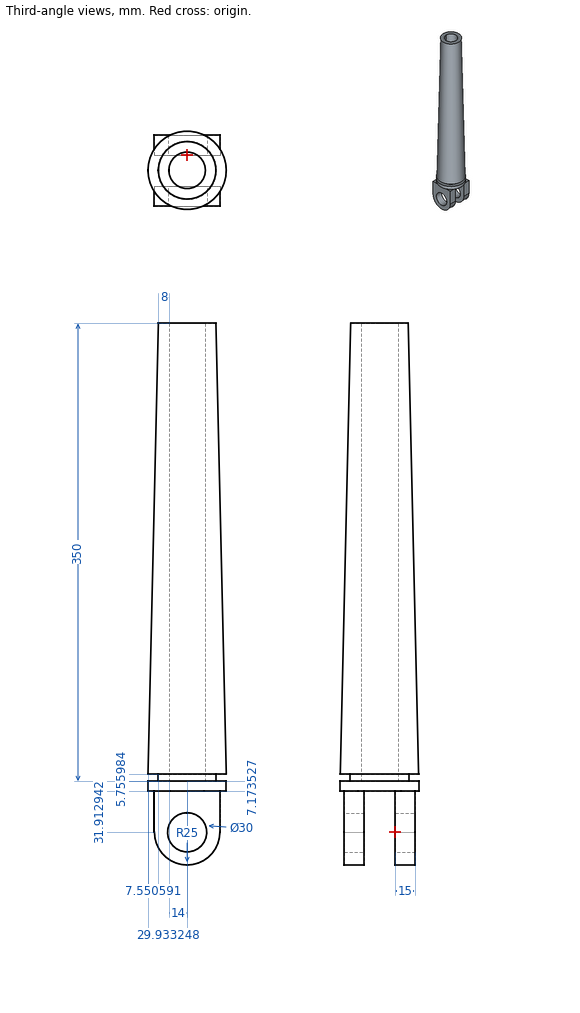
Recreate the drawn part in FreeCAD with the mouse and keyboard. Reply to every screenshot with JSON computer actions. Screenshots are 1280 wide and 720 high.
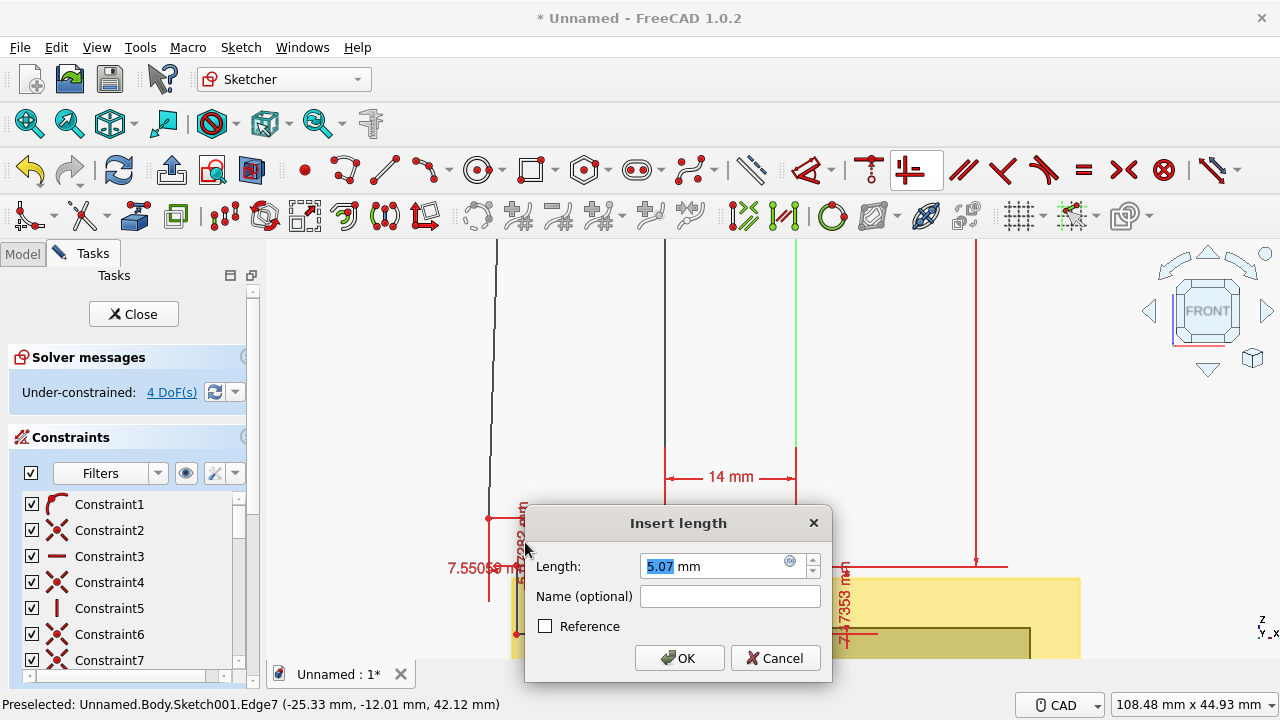
{"action": "type", "text": "5.755984"}
{"action": "key", "text": "Return"}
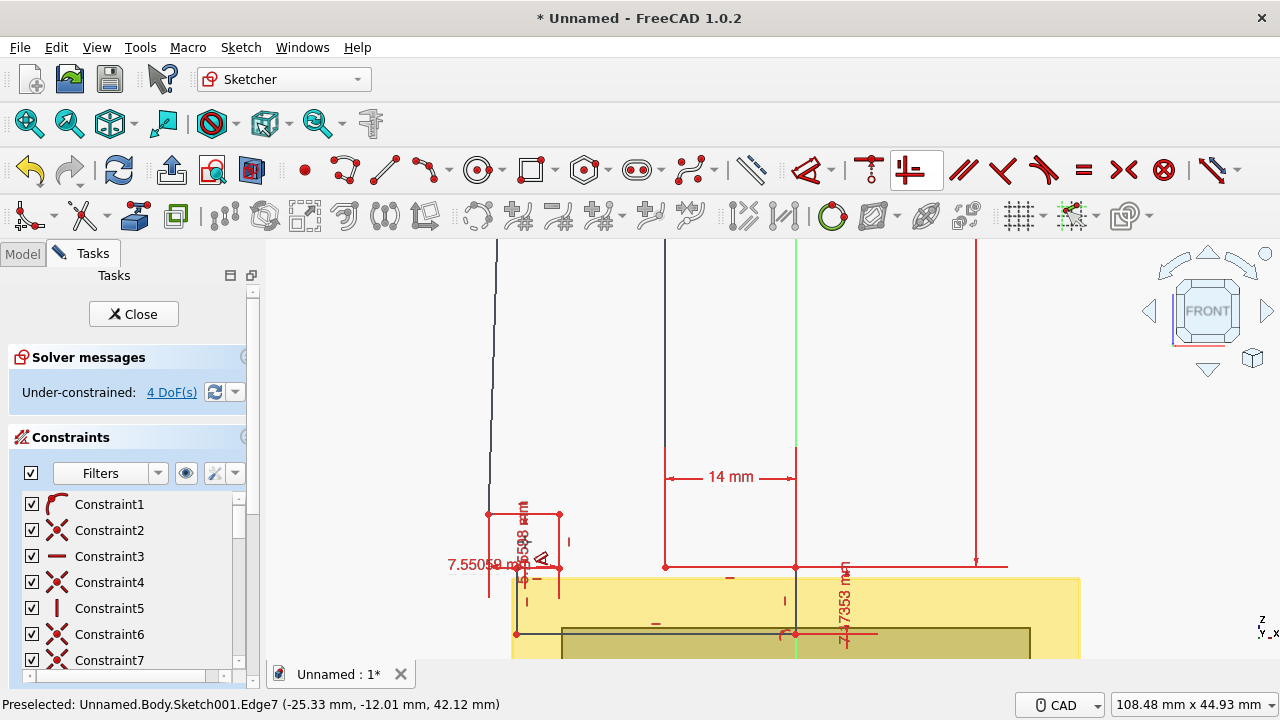
{"action": "left_click", "coordinate": [546, 568]}
{"action": "left_click", "coordinate": [538, 602]}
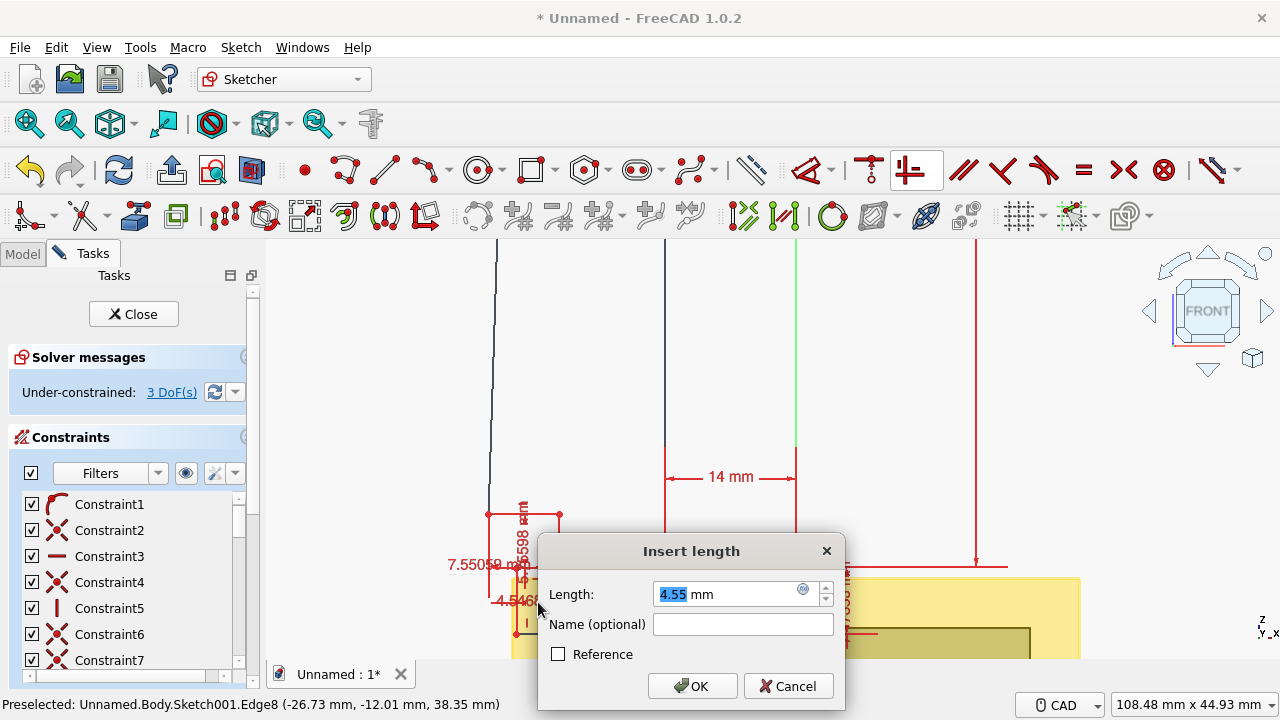
{"action": "type", "text": "7.550591"}
{"action": "key", "text": "Return"}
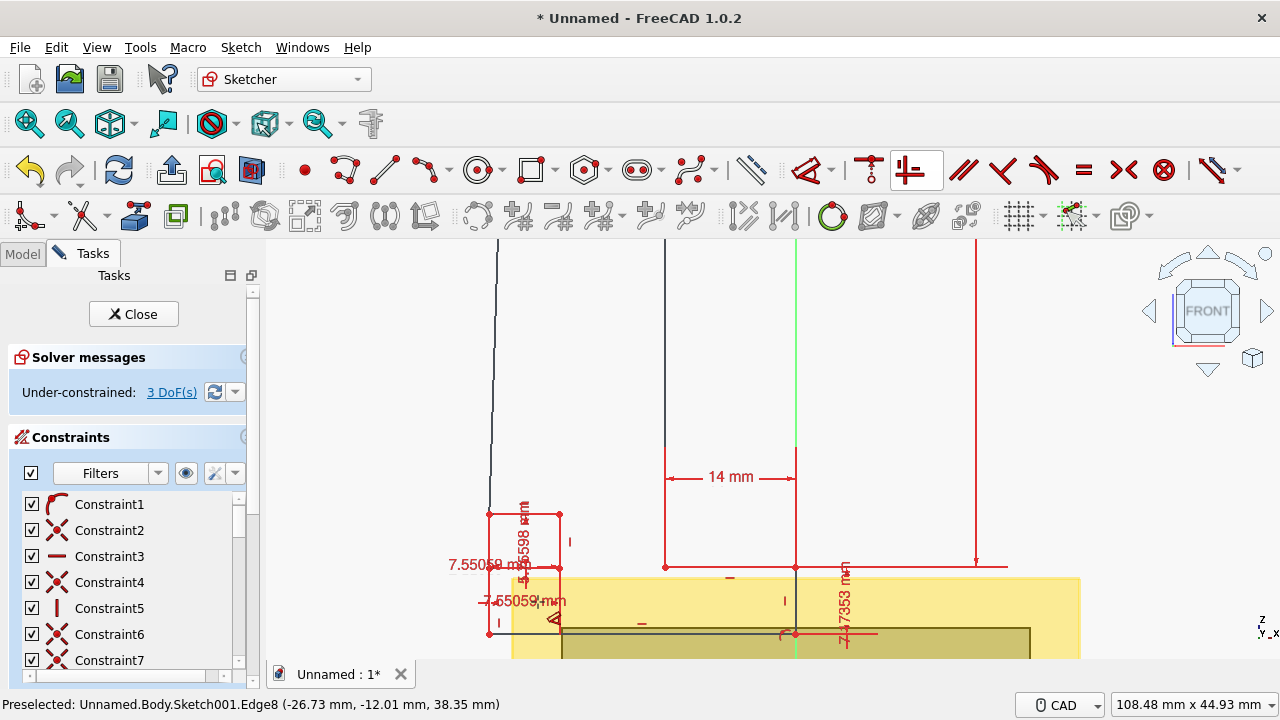
{"action": "left_click", "coordinate": [489, 588]}
{"action": "left_click", "coordinate": [455, 600]}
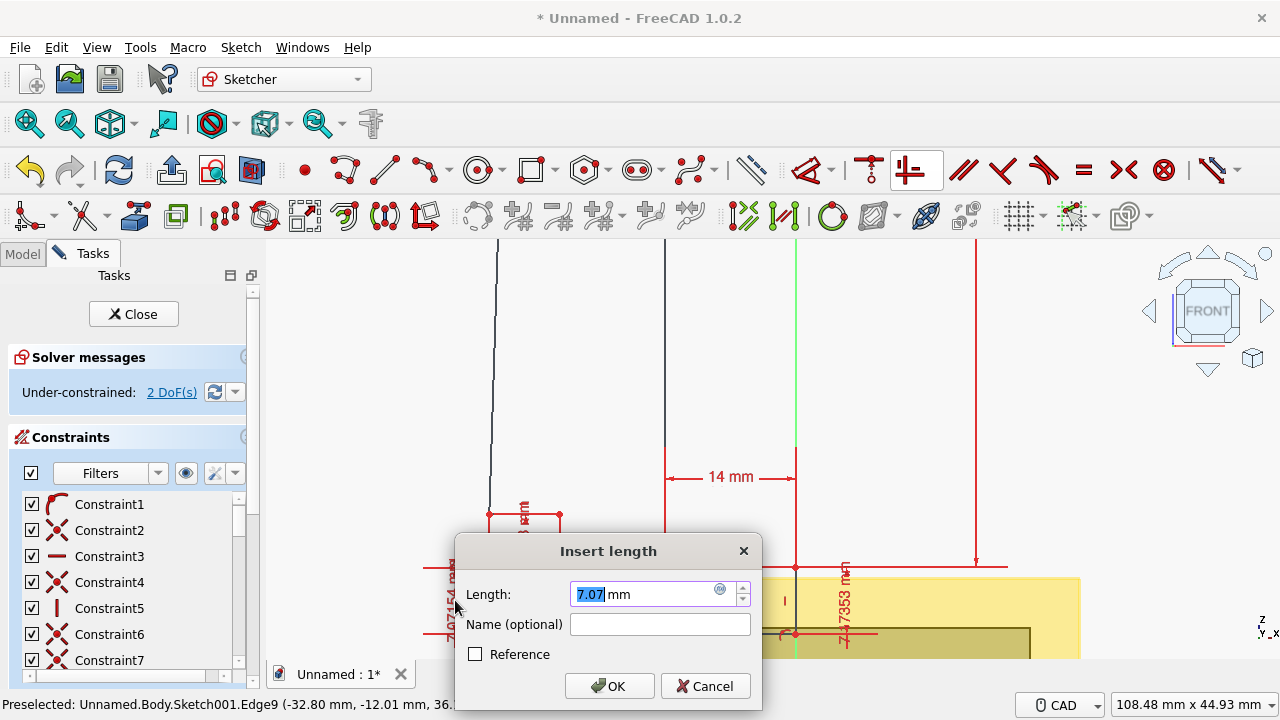
{"action": "type", "text": "7.173527"}
{"action": "key", "text": "Return"}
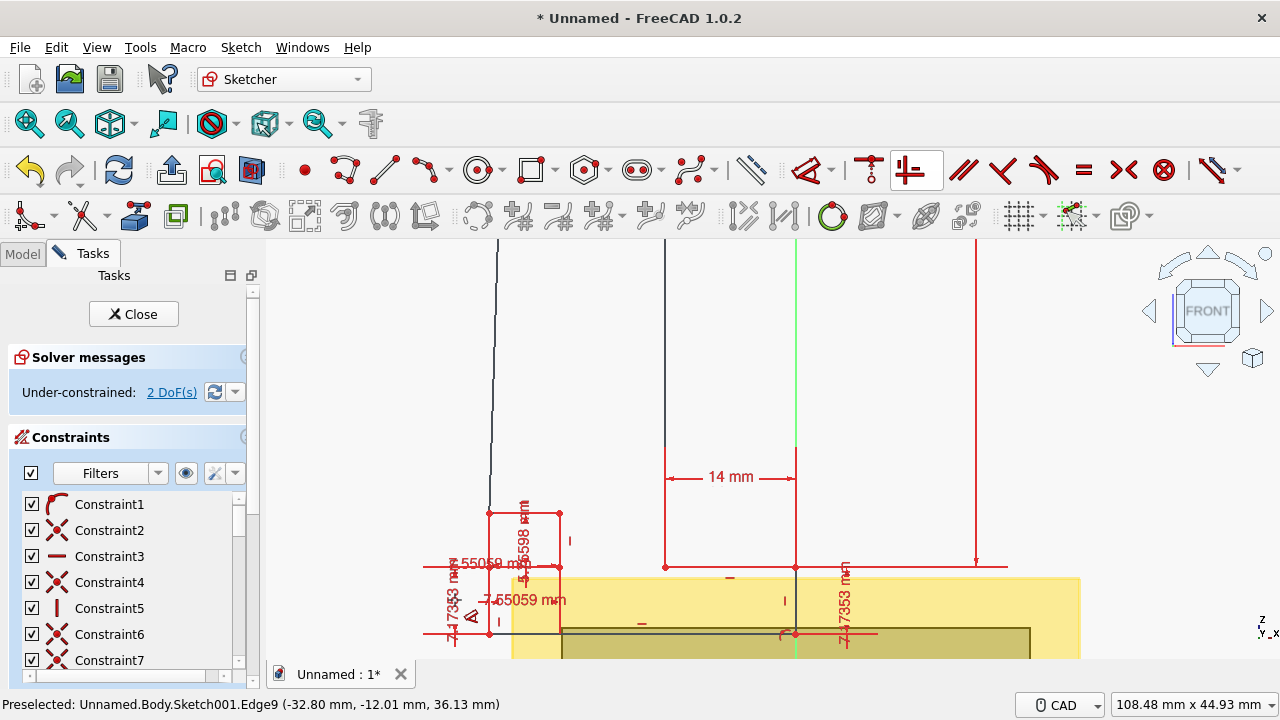
{"action": "scroll", "coordinate": [708, 557], "scroll_direction": "down", "scroll_amount": 13}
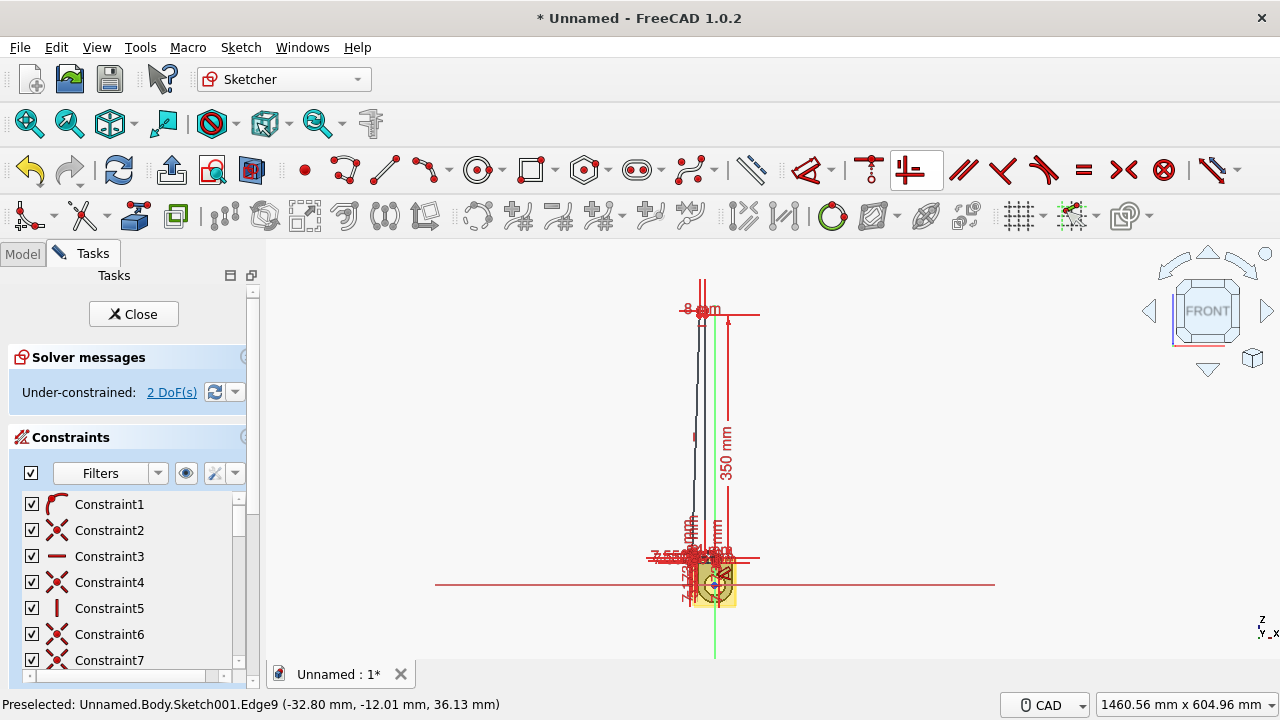
{"action": "scroll", "coordinate": [699, 563], "scroll_direction": "up", "scroll_amount": 5}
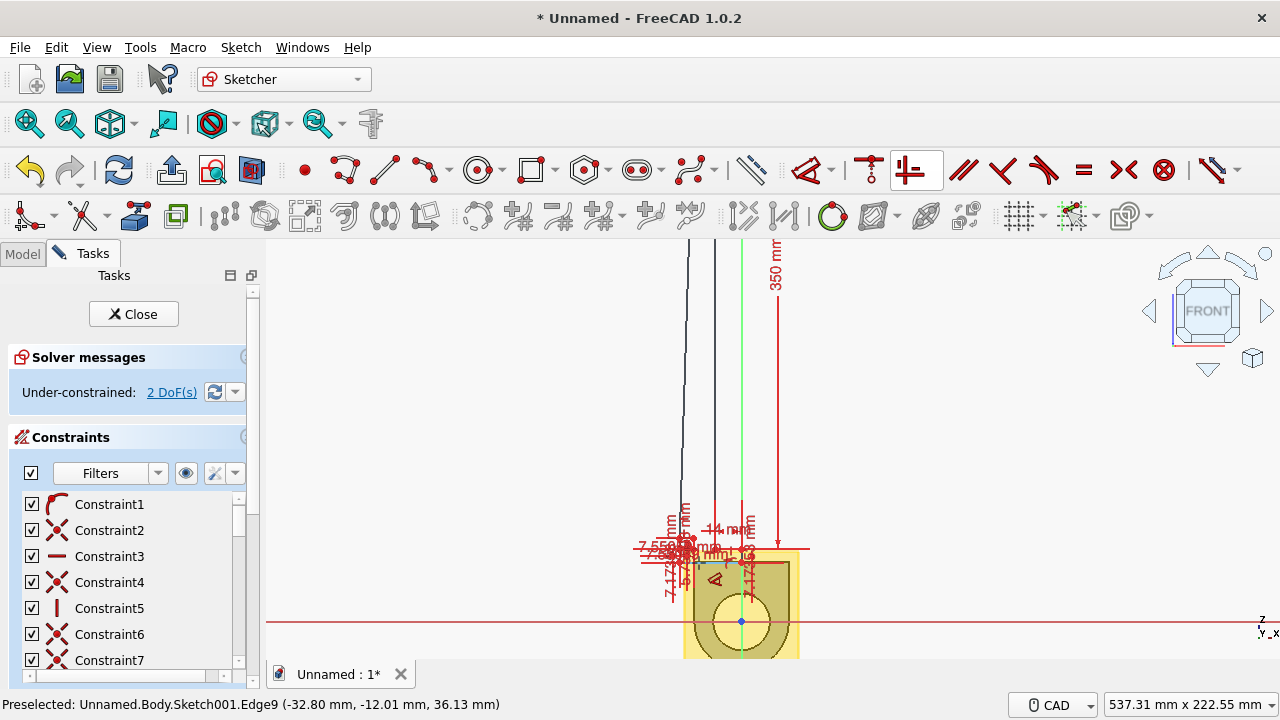
{"action": "left_click", "coordinate": [698, 563]}
{"action": "left_click", "coordinate": [711, 597]}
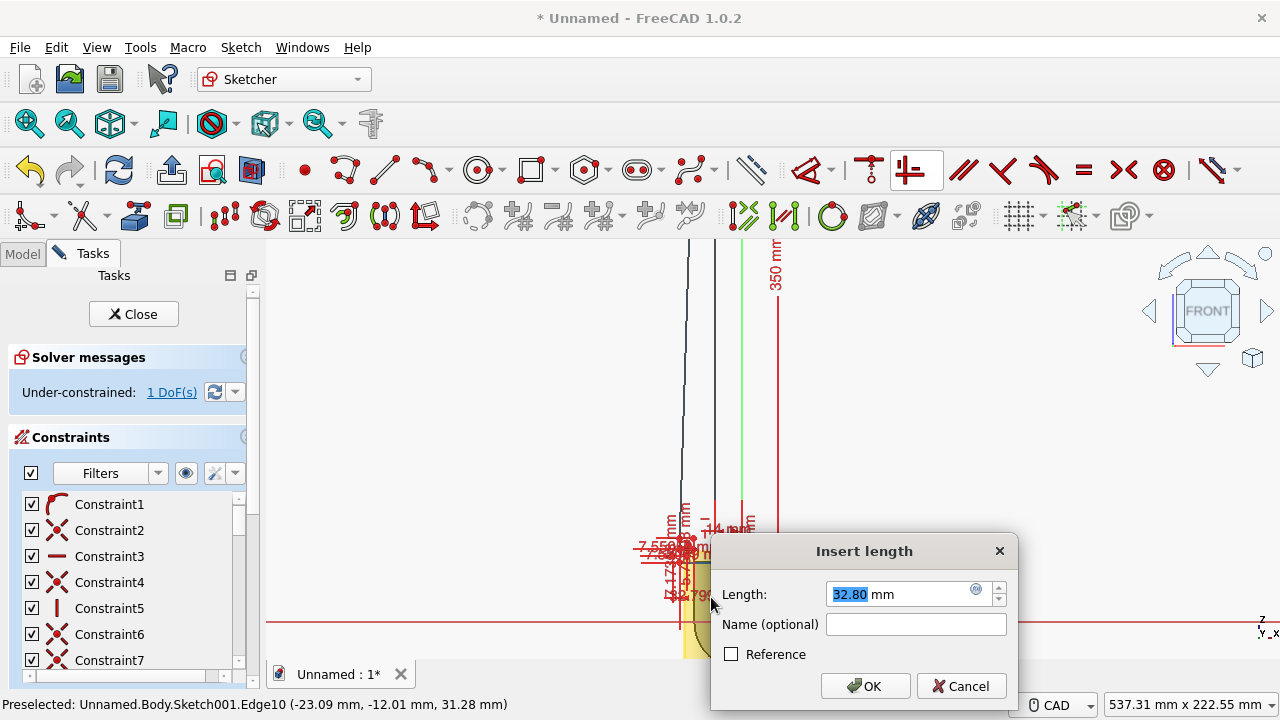
{"action": "type", "text": "29.933248"}
{"action": "key", "text": "Return"}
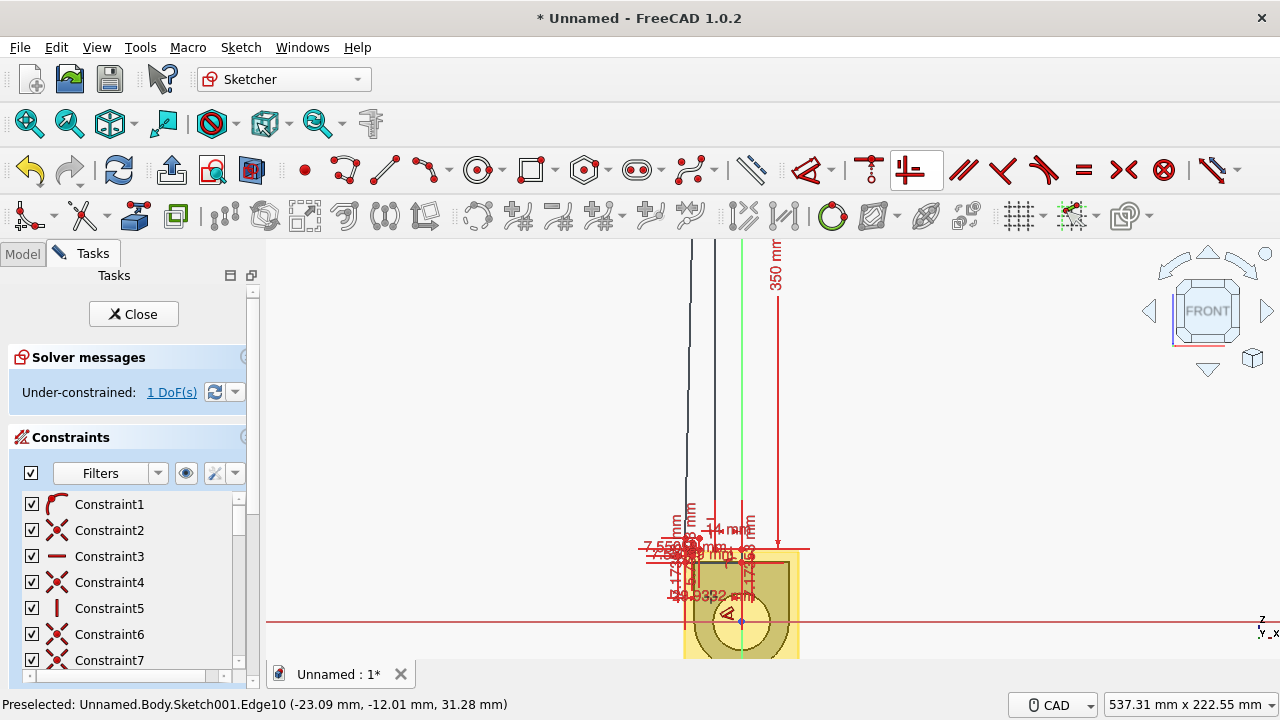
{"action": "left_click", "coordinate": [742, 563]}
{"action": "left_click", "coordinate": [800, 592]}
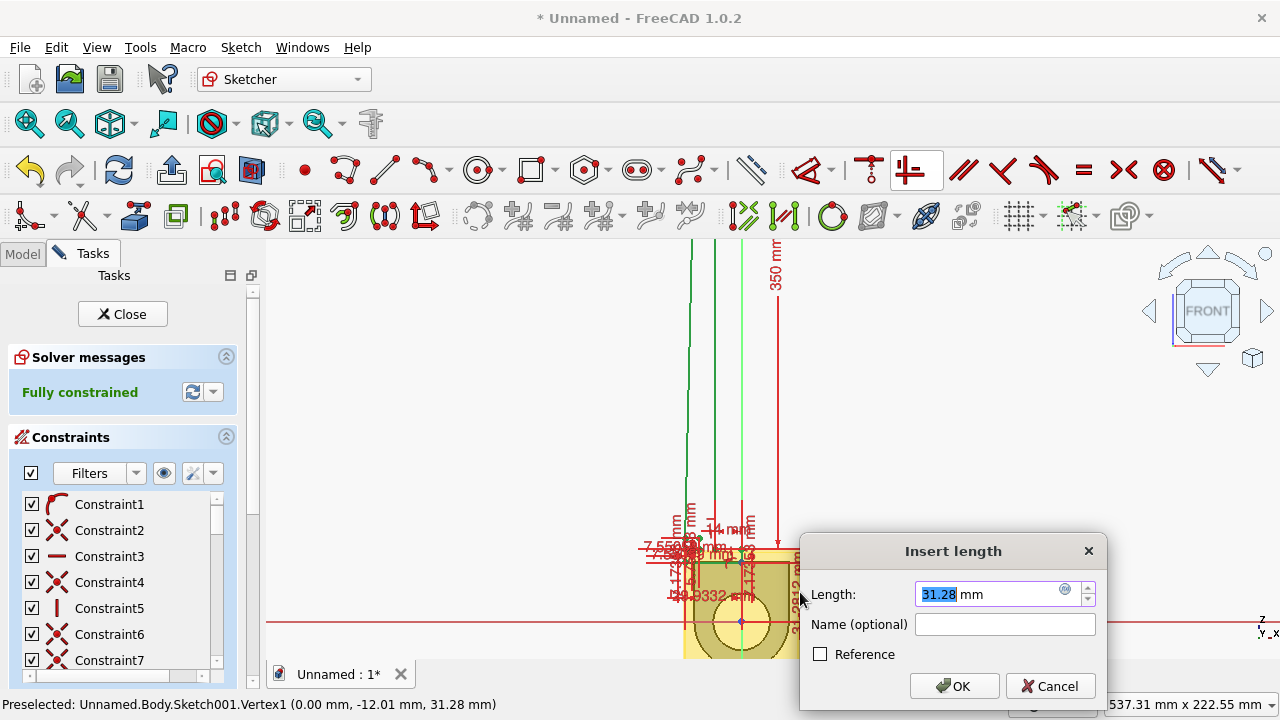
{"action": "type", "text": "31.912942"}
{"action": "key", "text": "Return"}
{"action": "key", "text": "Escape"}